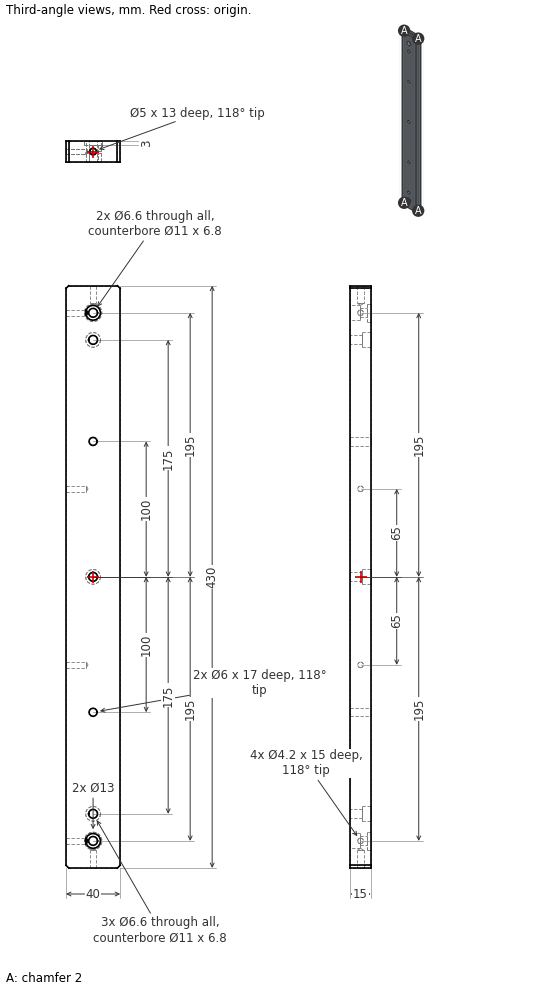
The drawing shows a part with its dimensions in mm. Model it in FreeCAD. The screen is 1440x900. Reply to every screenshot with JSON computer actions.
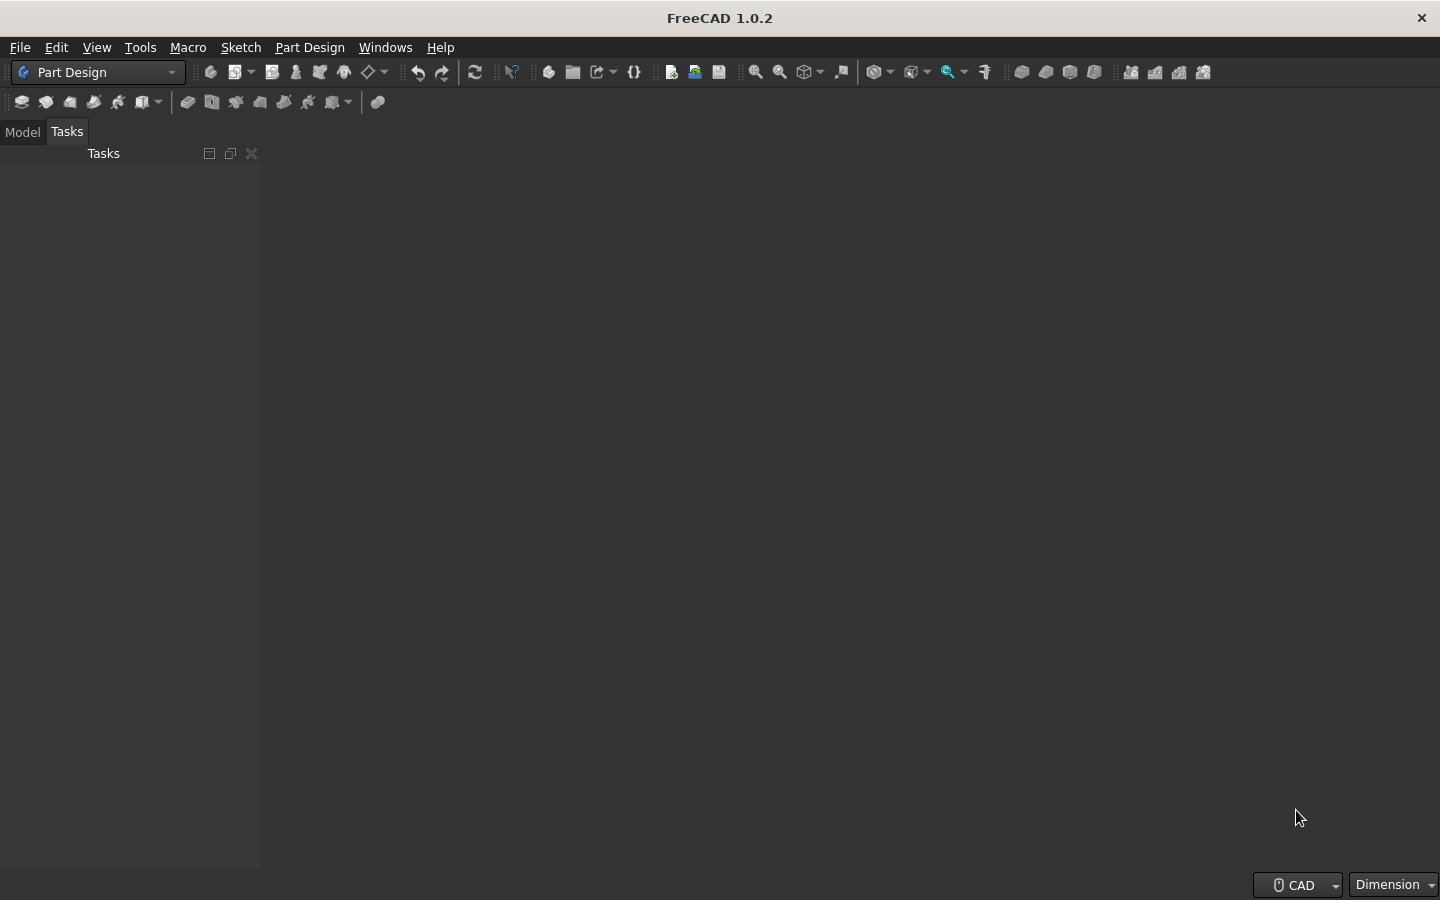
{"action": "key", "text": "ctrl+n"}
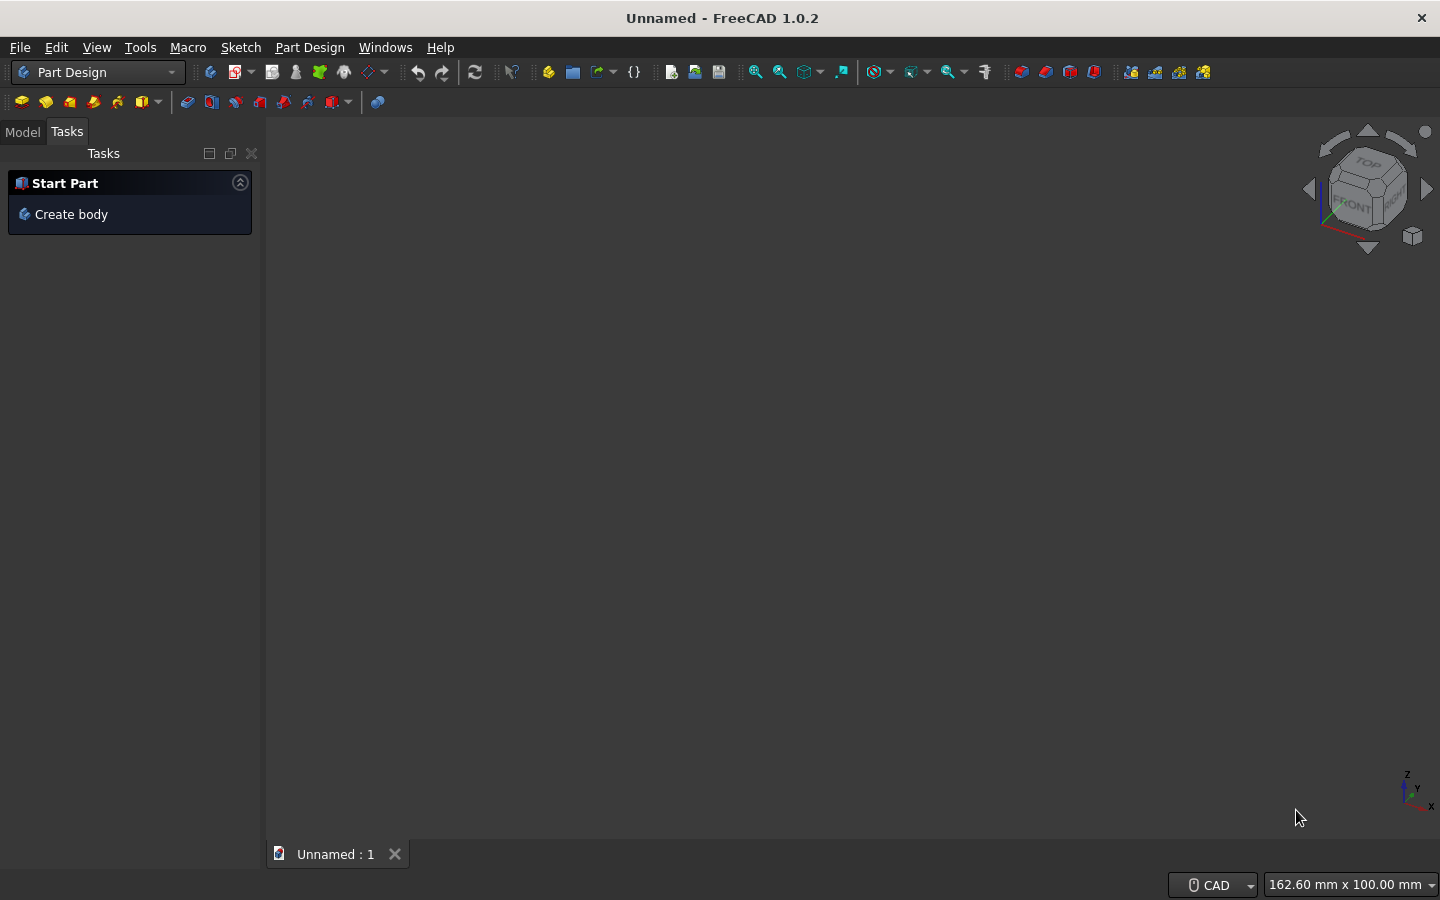
{"action": "left_click", "coordinate": [236, 72]}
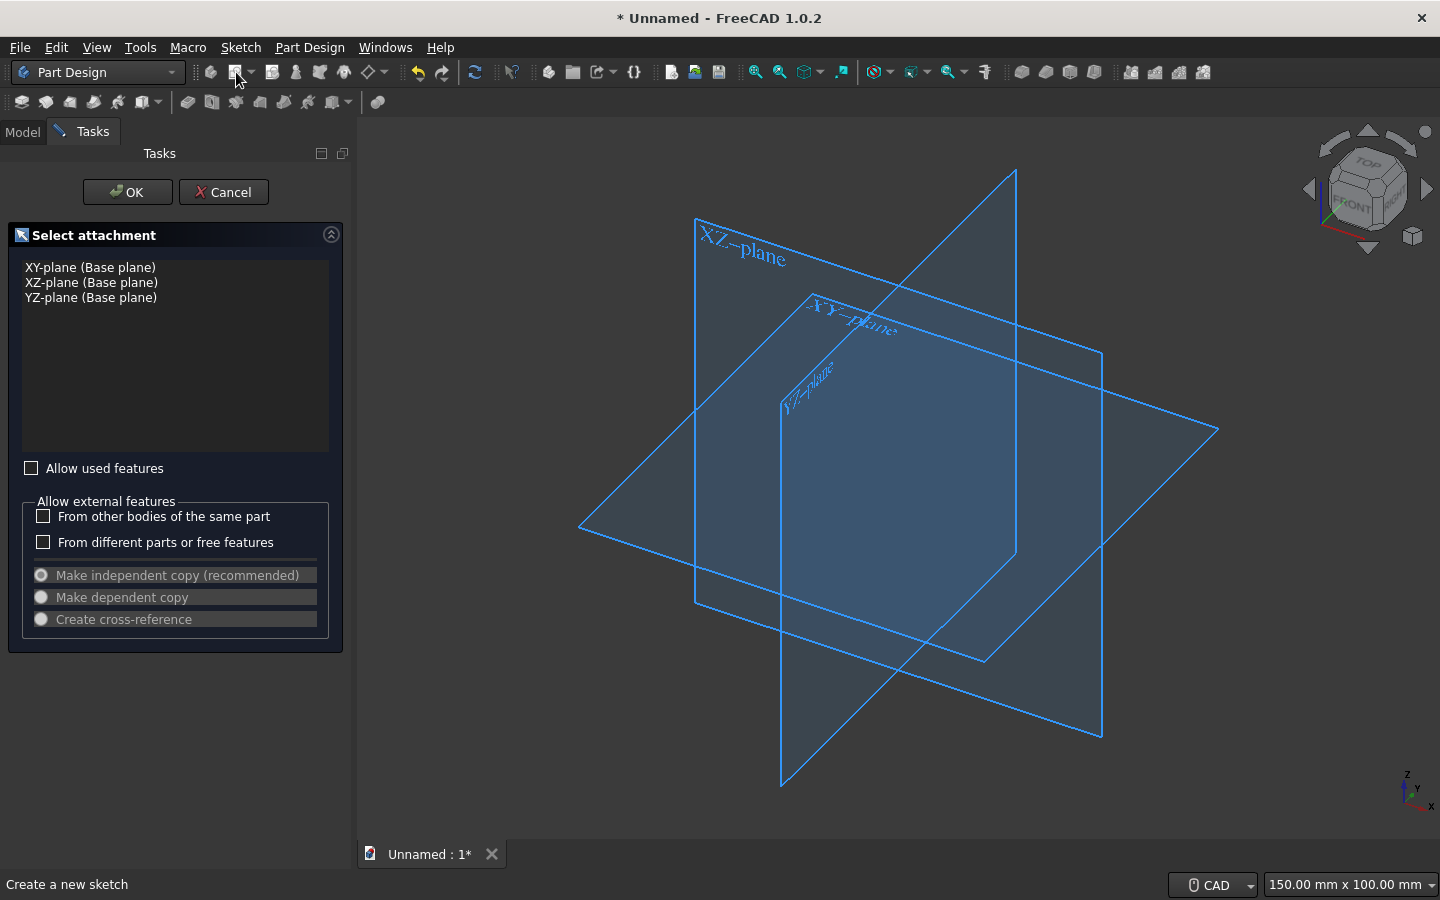
{"action": "left_click", "coordinate": [82, 282]}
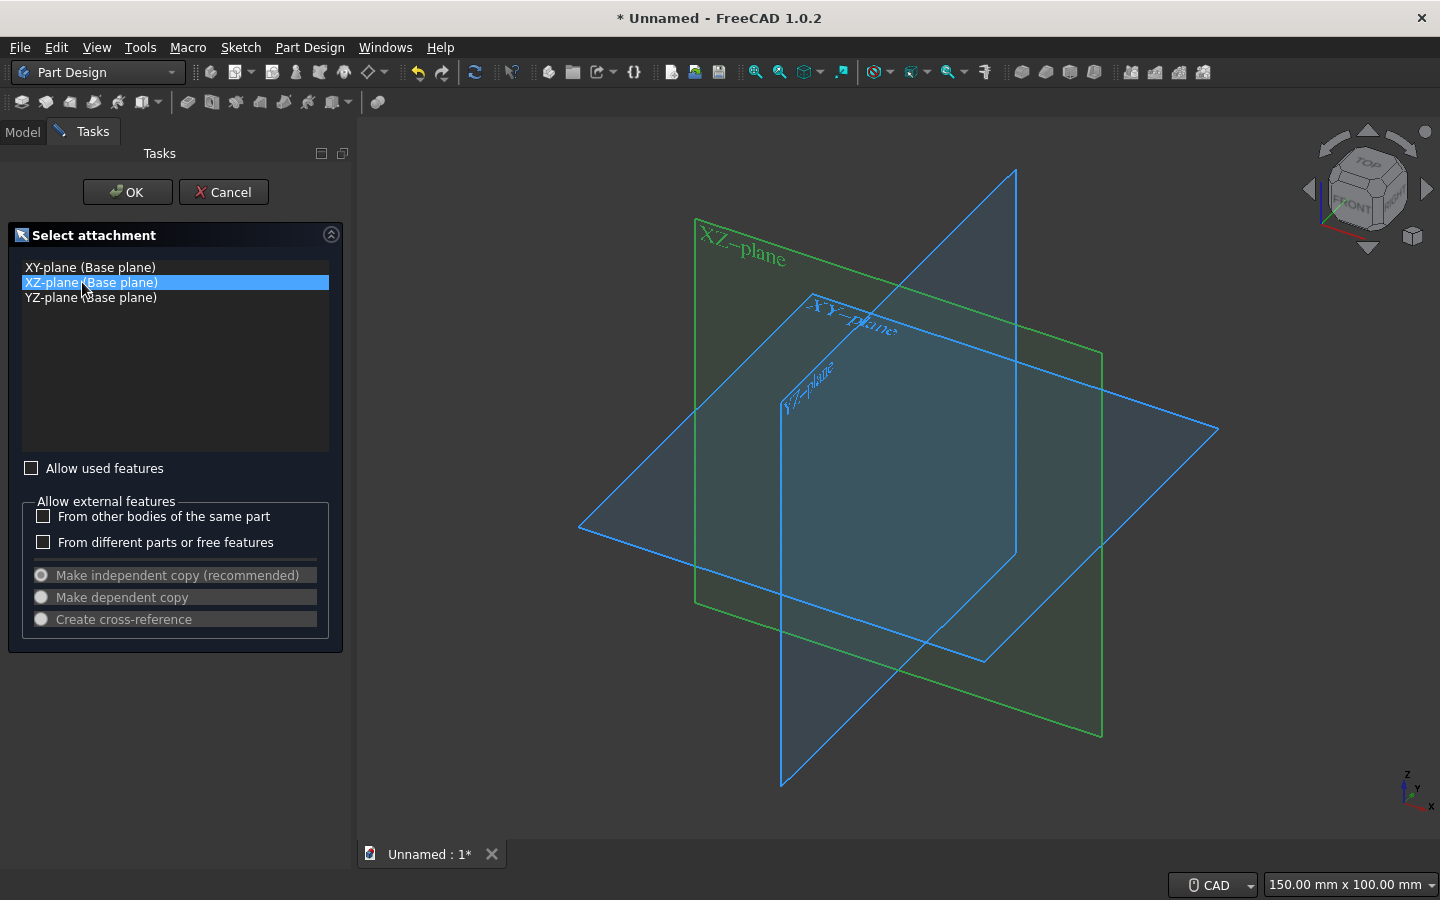
{"action": "left_click", "coordinate": [128, 192]}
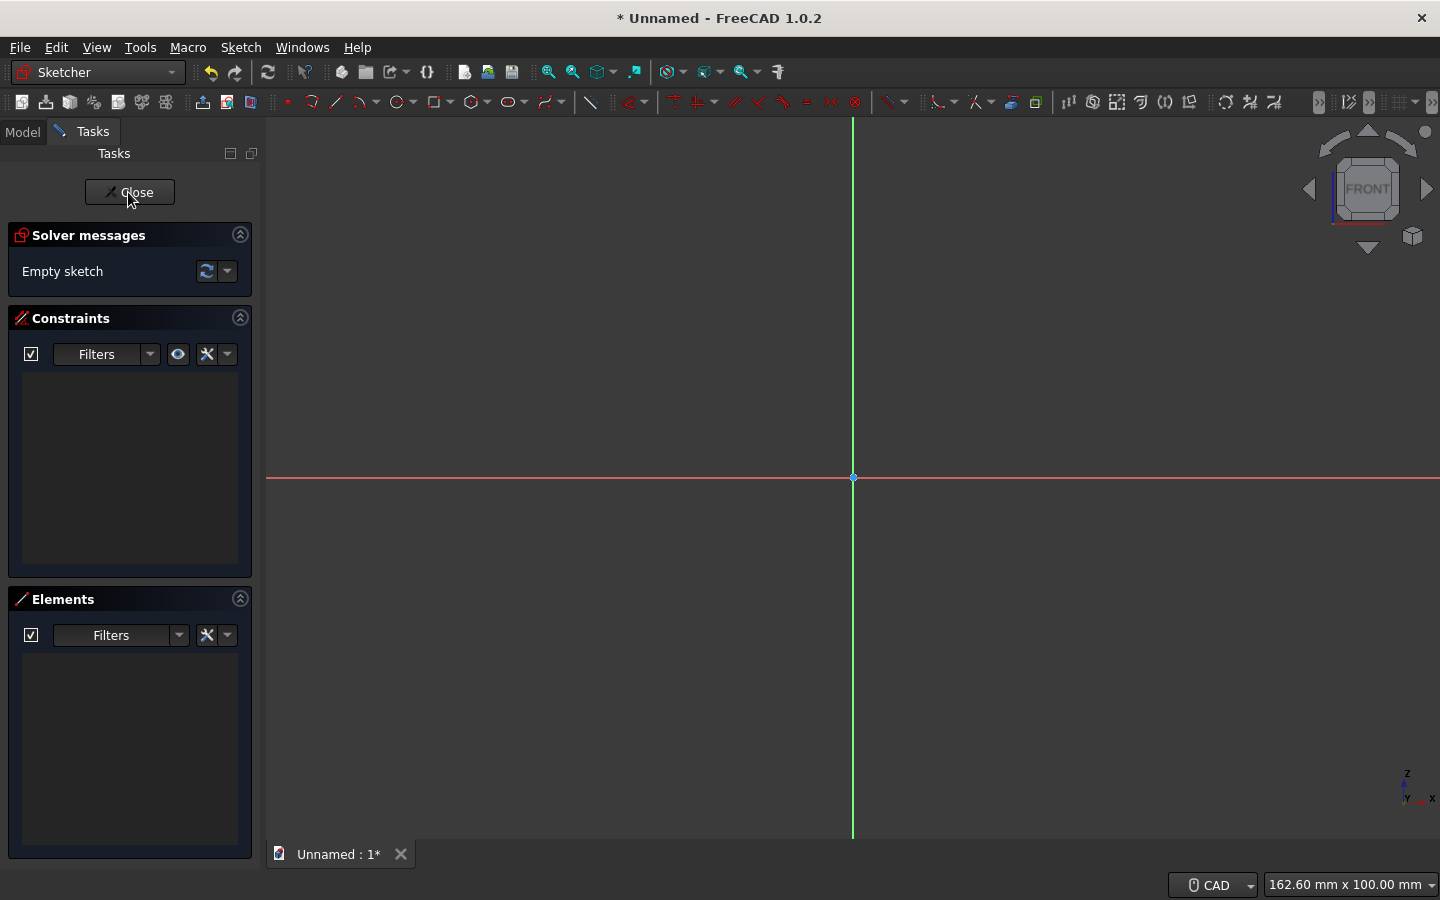
{"action": "scroll", "coordinate": [771, 478], "scroll_direction": "down", "scroll_amount": 9}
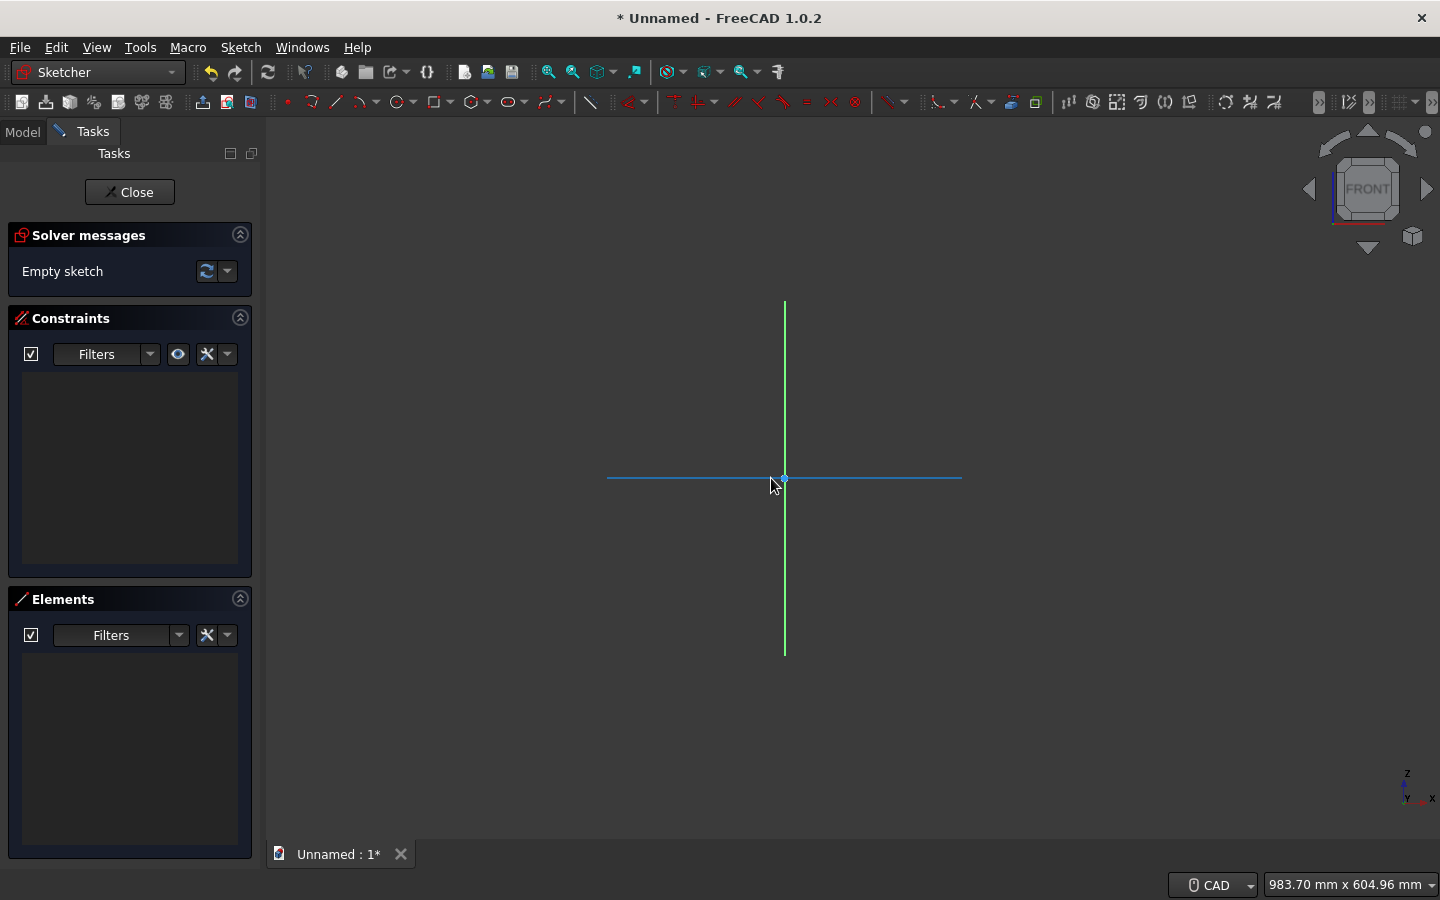
{"action": "left_click", "coordinate": [452, 102]}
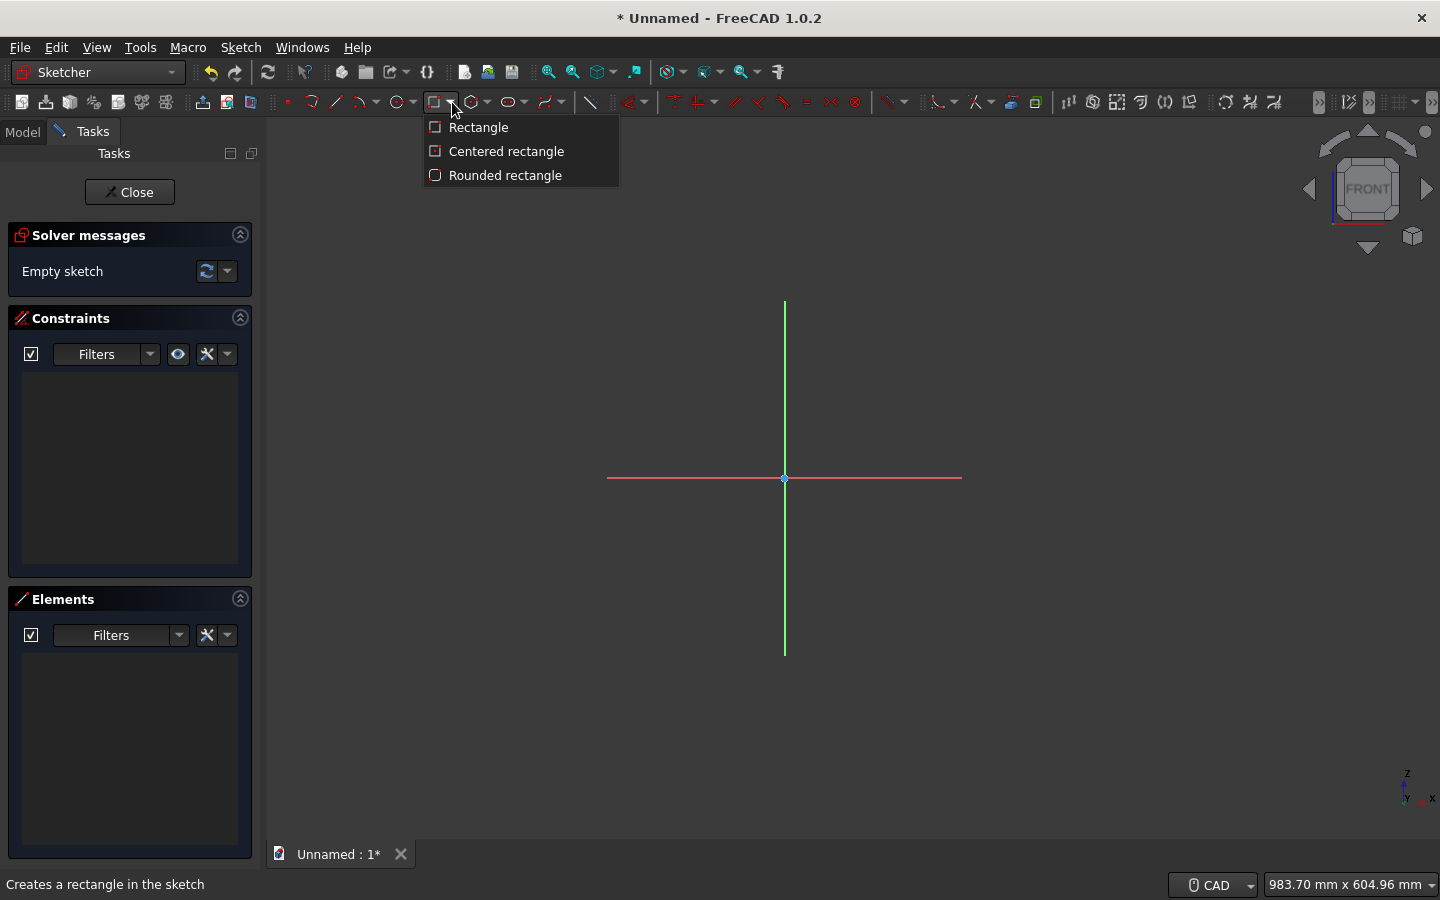
{"action": "left_click", "coordinate": [522, 151]}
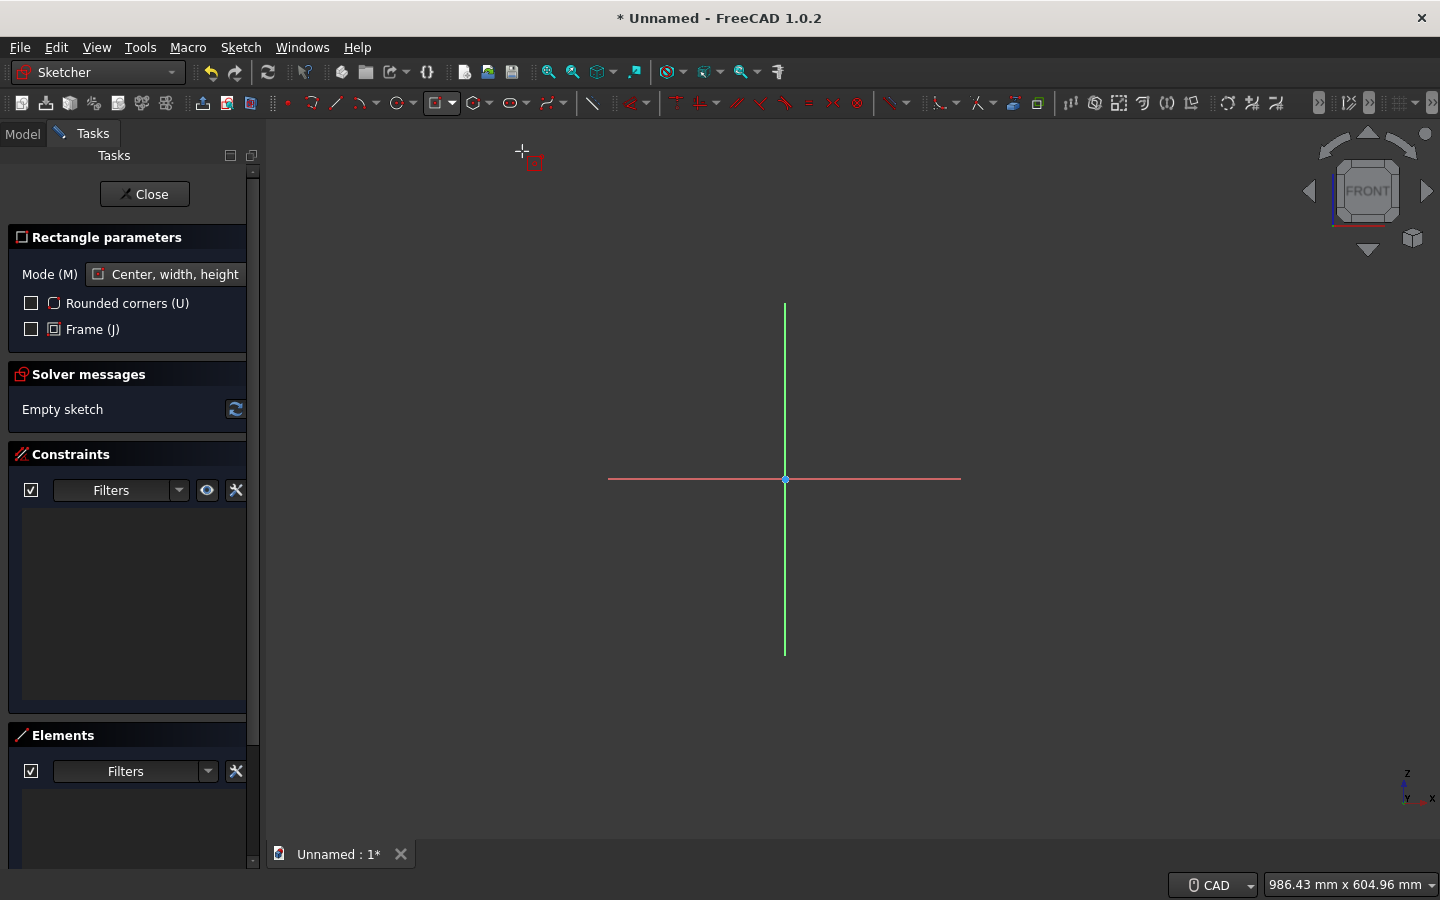
{"action": "left_click", "coordinate": [785, 479]}
{"action": "left_click", "coordinate": [809, 224]}
{"action": "key", "text": "Escape"}